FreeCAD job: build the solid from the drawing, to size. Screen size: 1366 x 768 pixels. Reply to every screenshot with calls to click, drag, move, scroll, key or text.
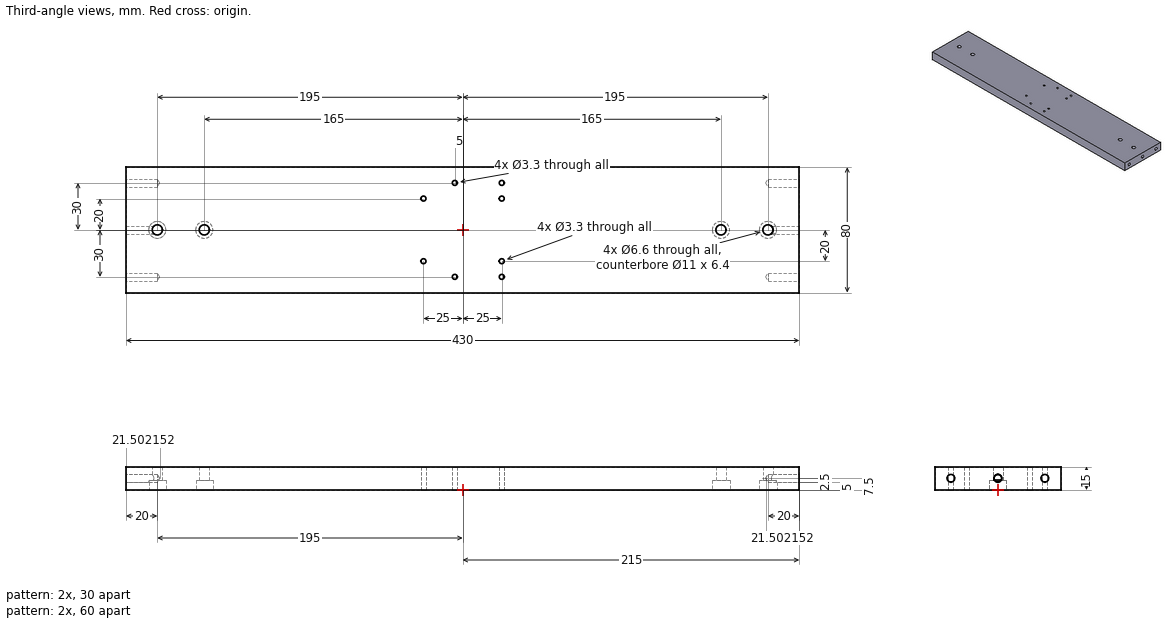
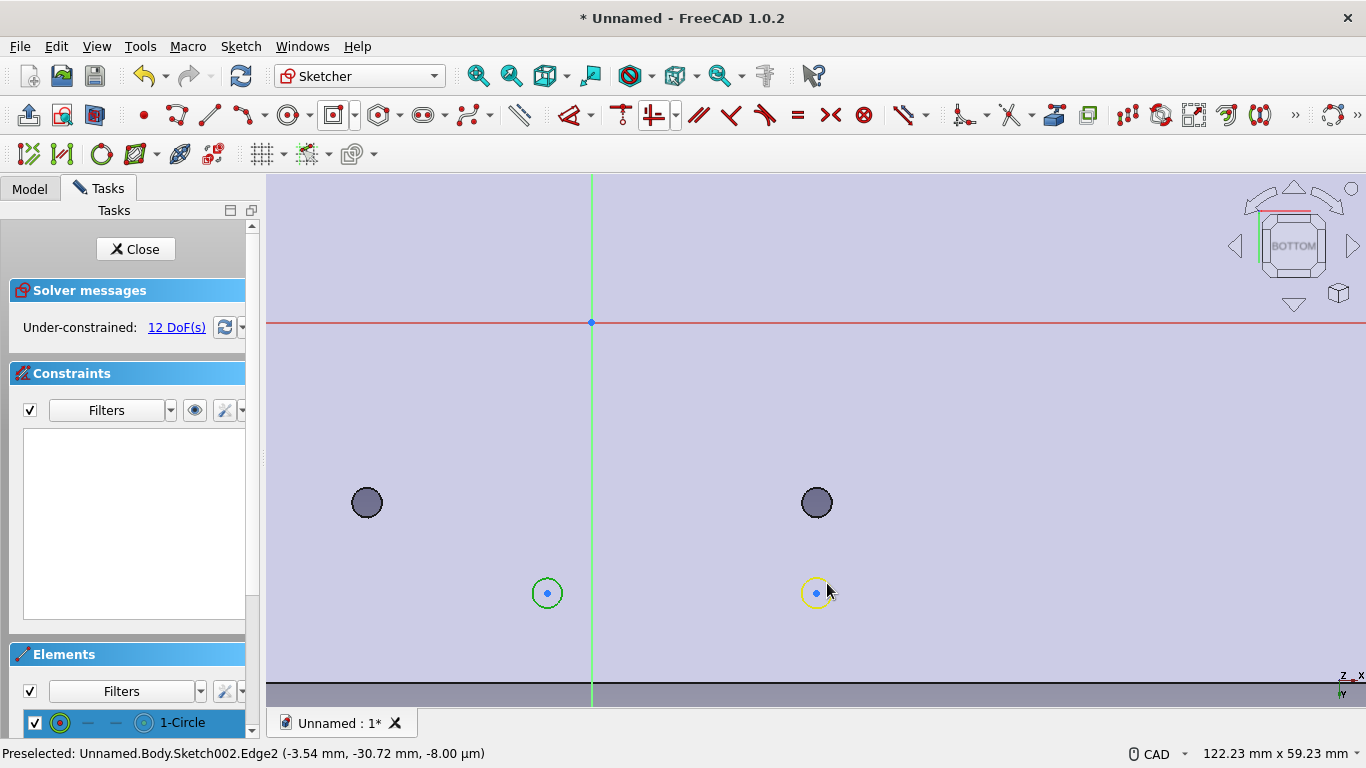
click(827, 582)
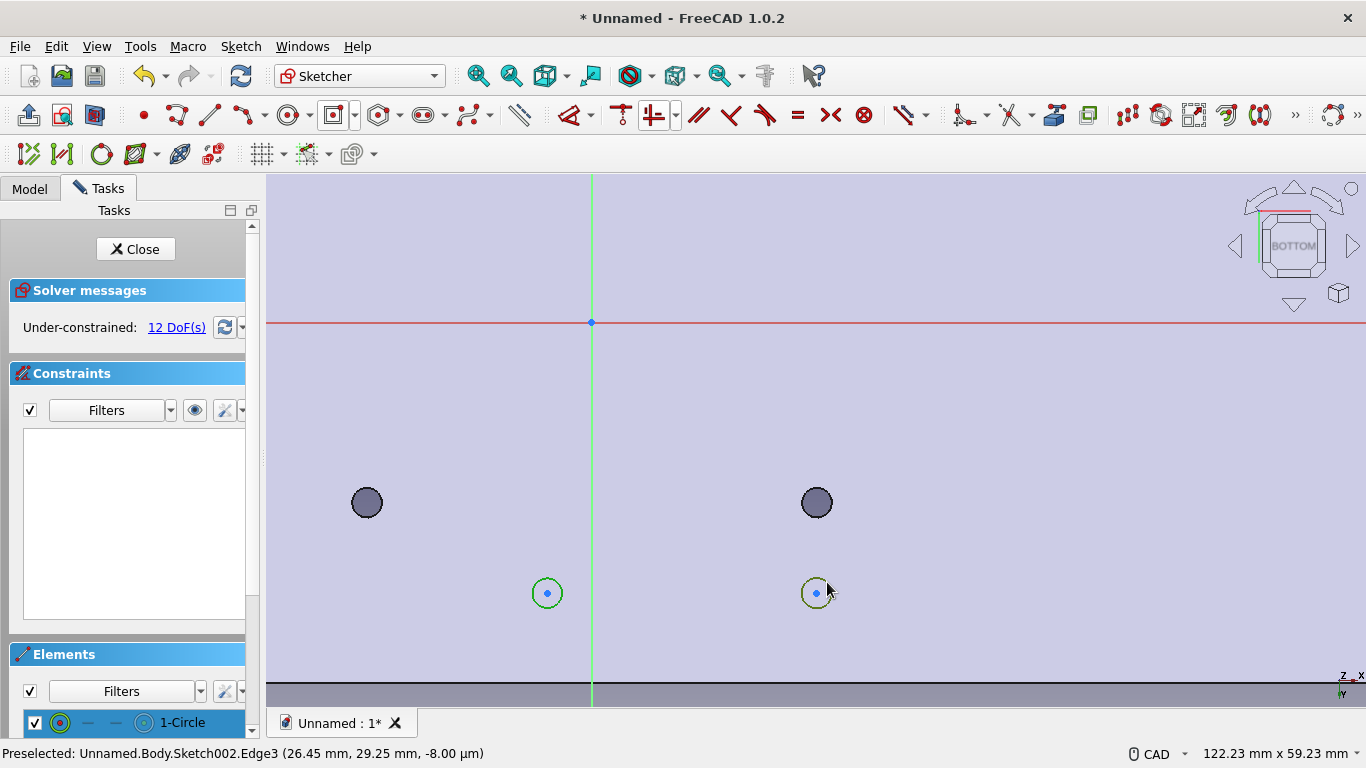
scroll(827, 584, down, 3)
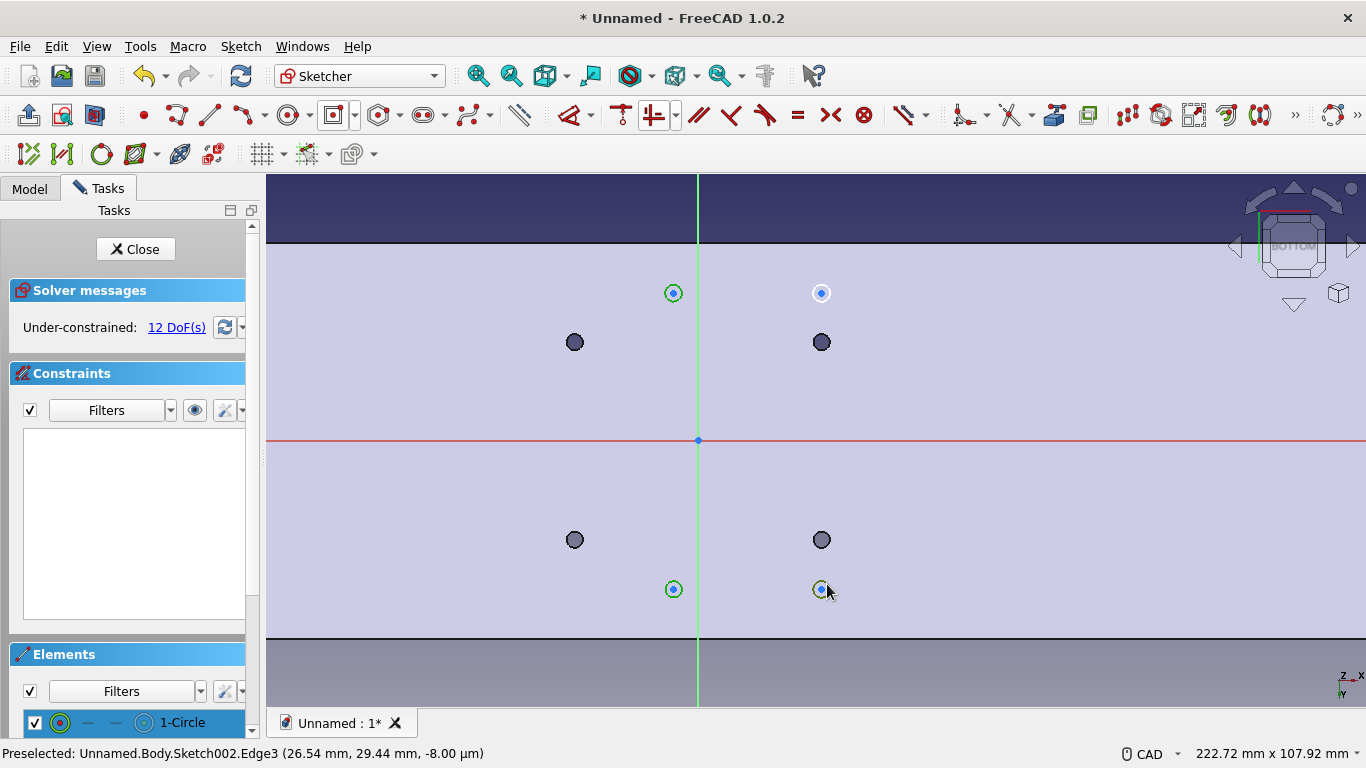
scroll(828, 287, up, 3)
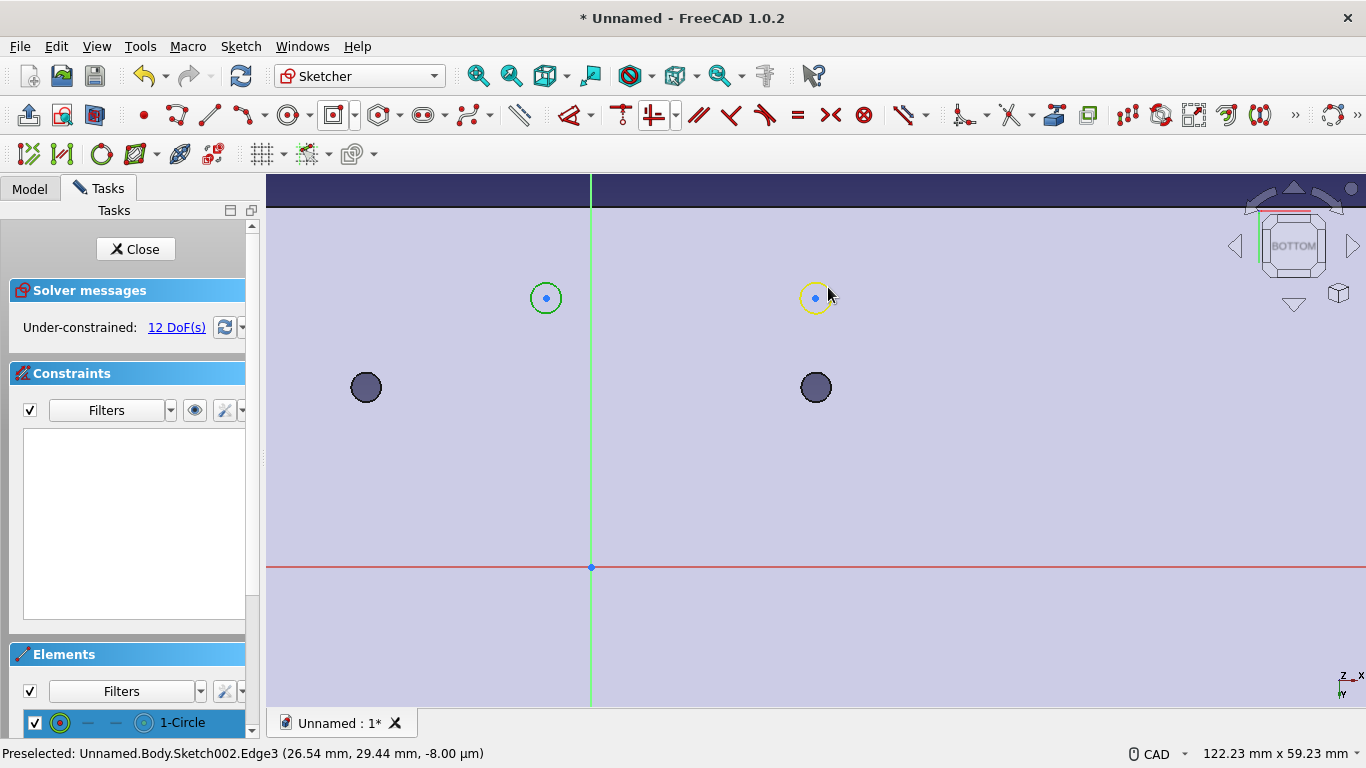
click(827, 287)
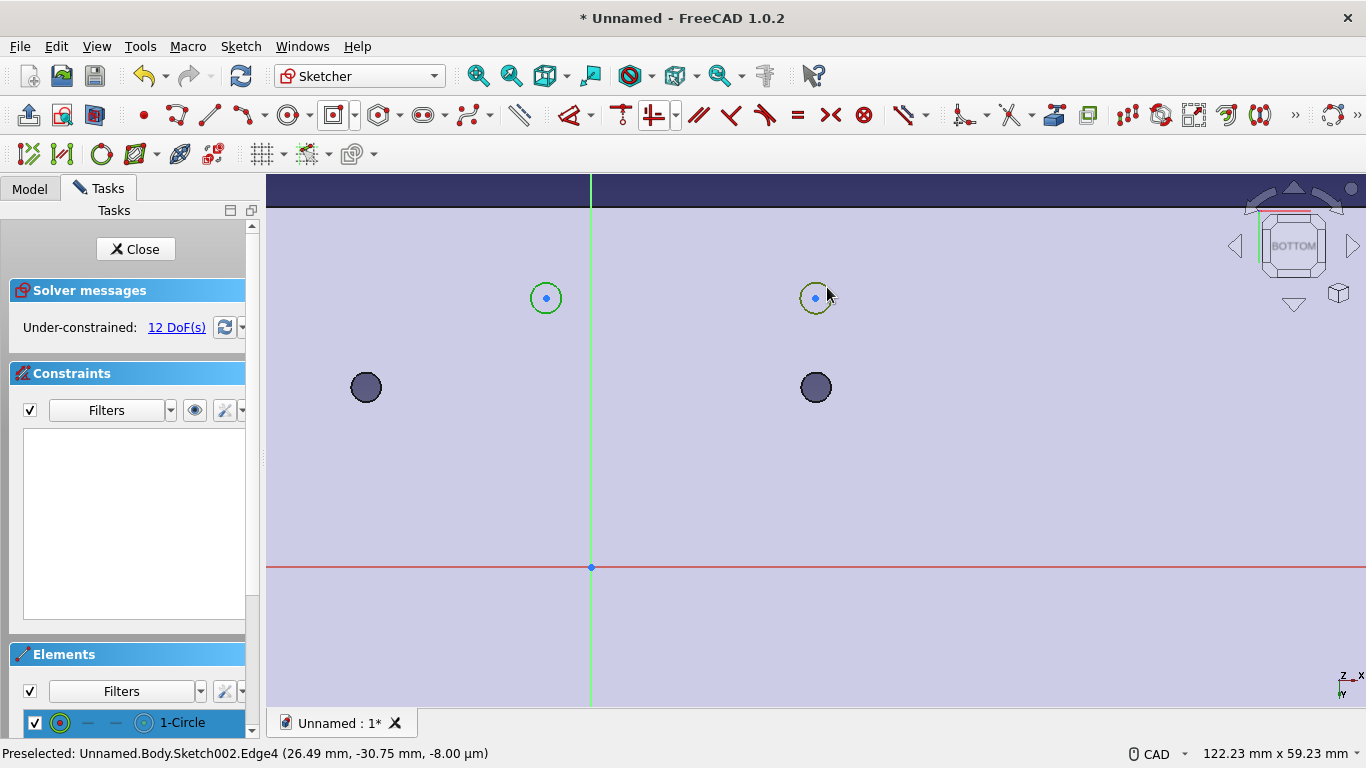
click(798, 116)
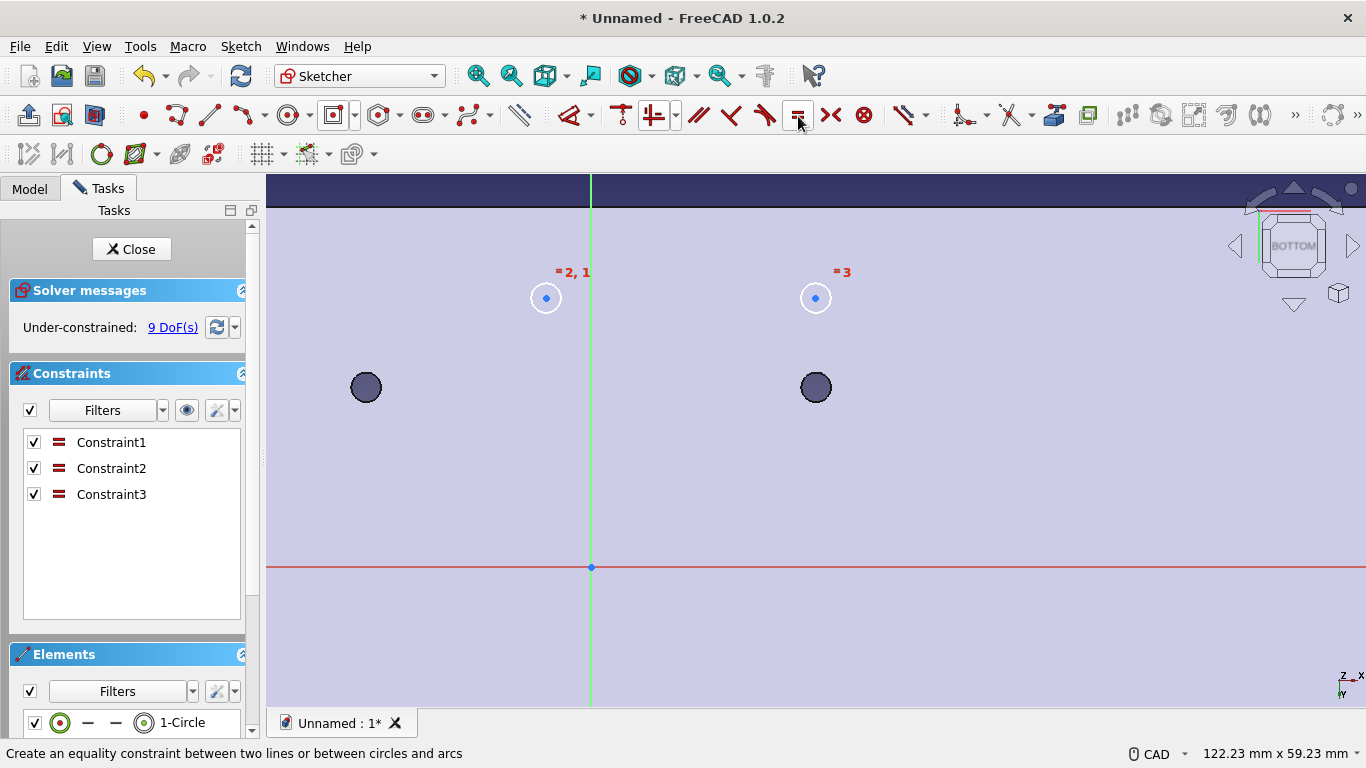
scroll(828, 286, down, 3)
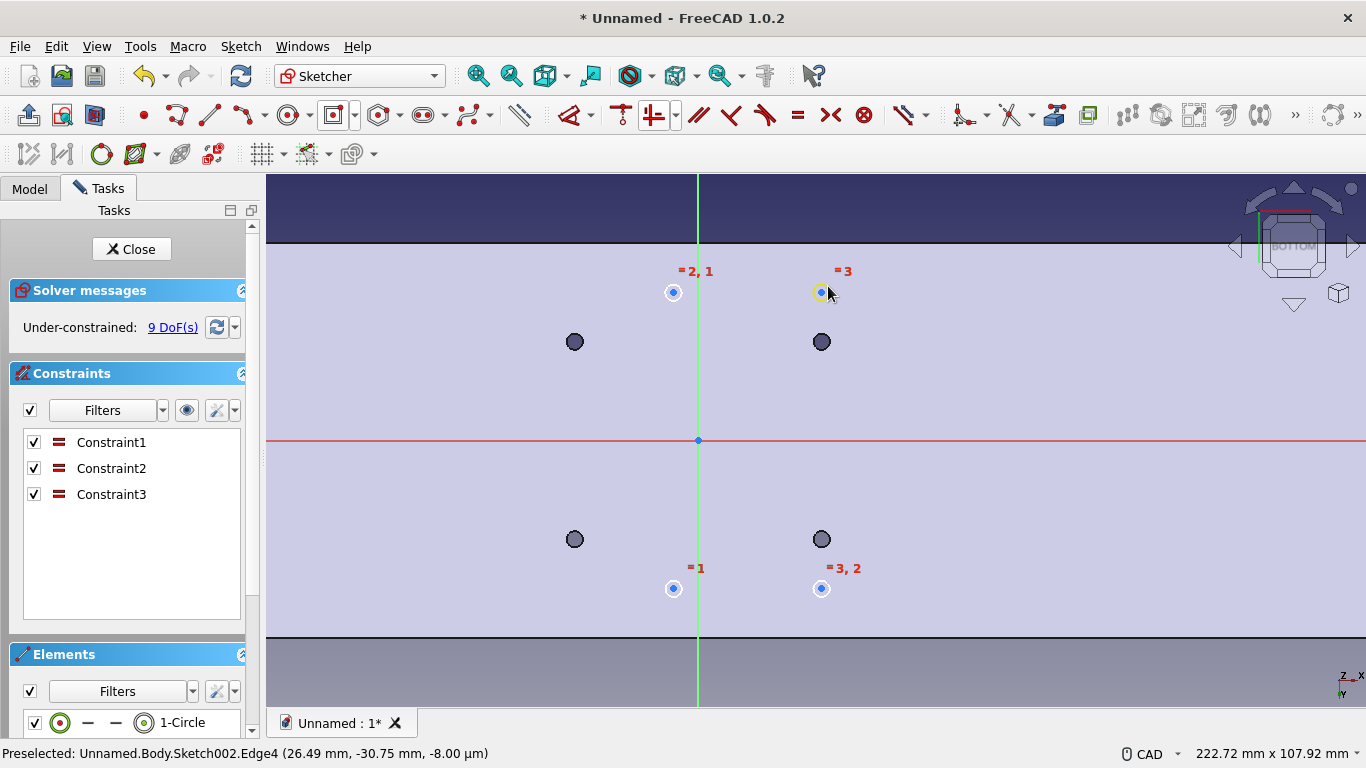
click(674, 589)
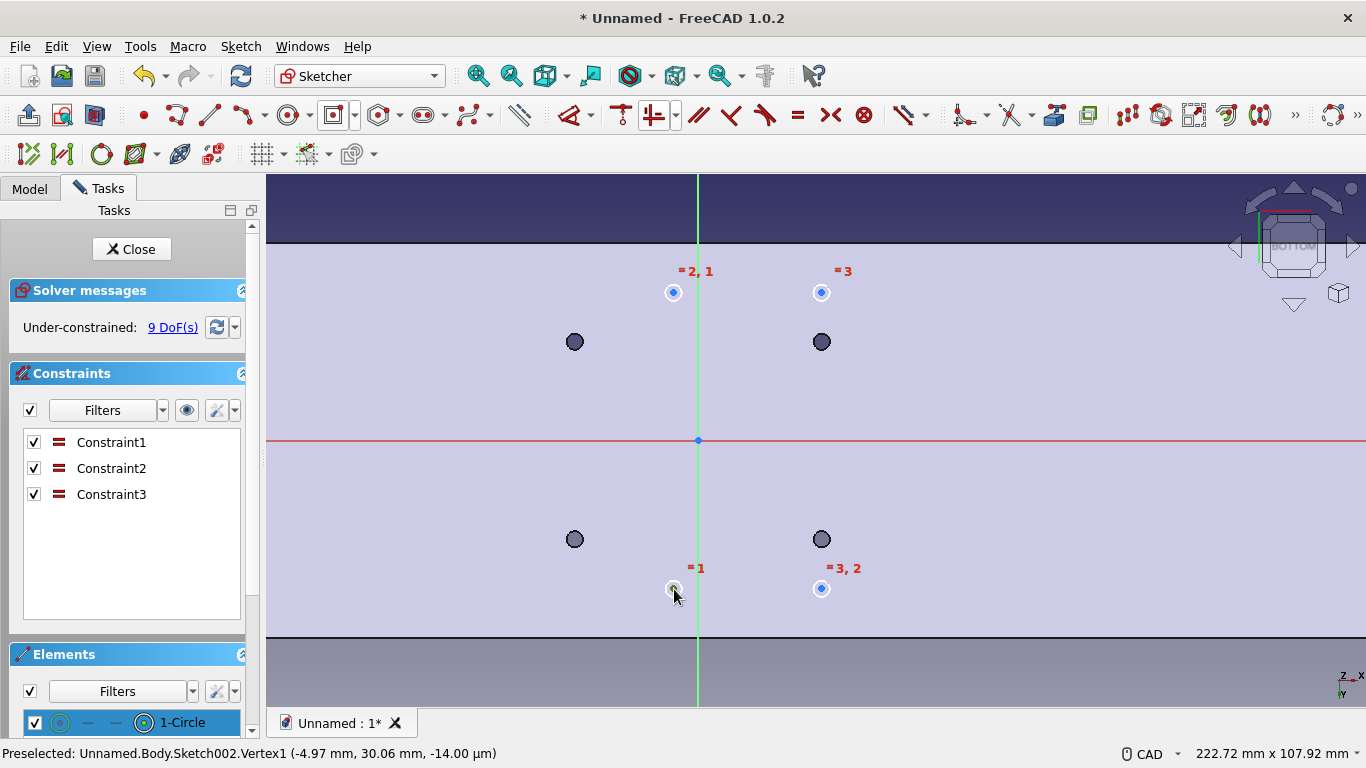
click(674, 293)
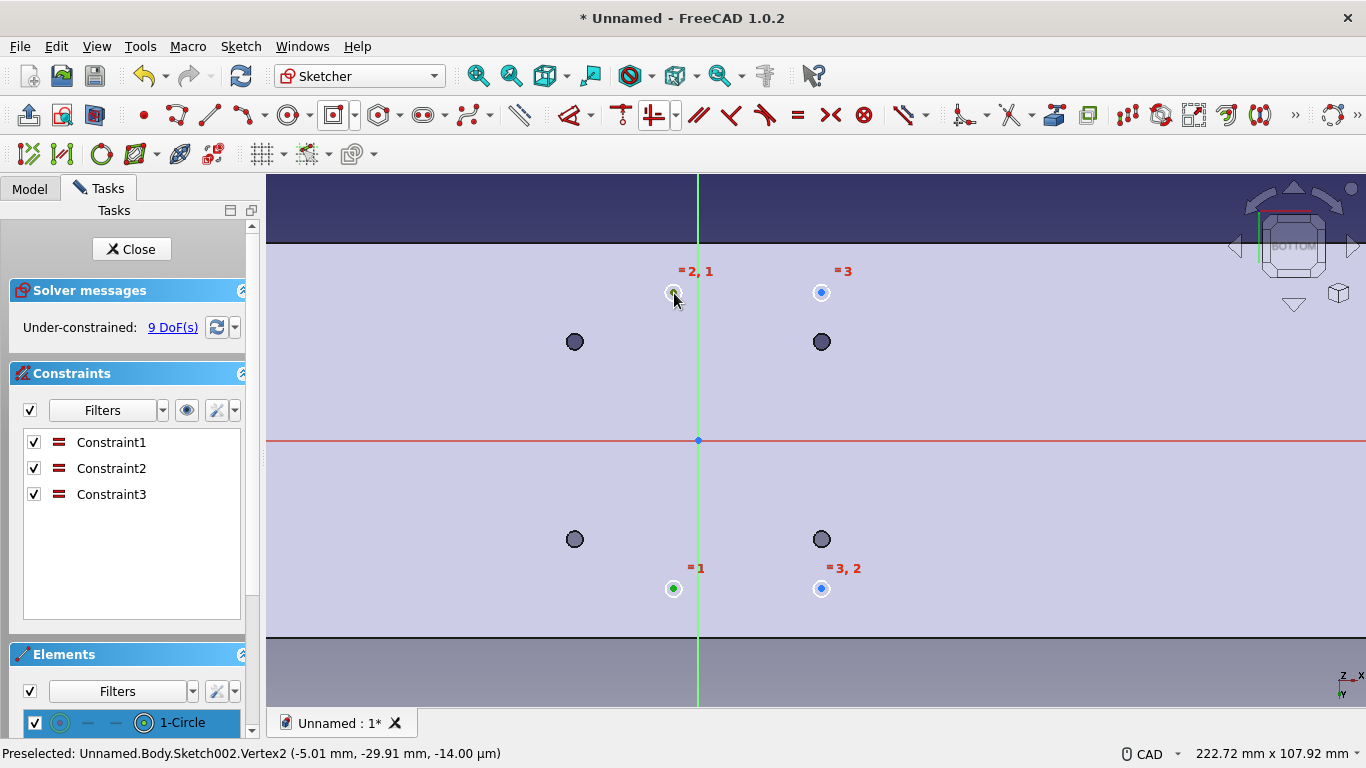
click(676, 116)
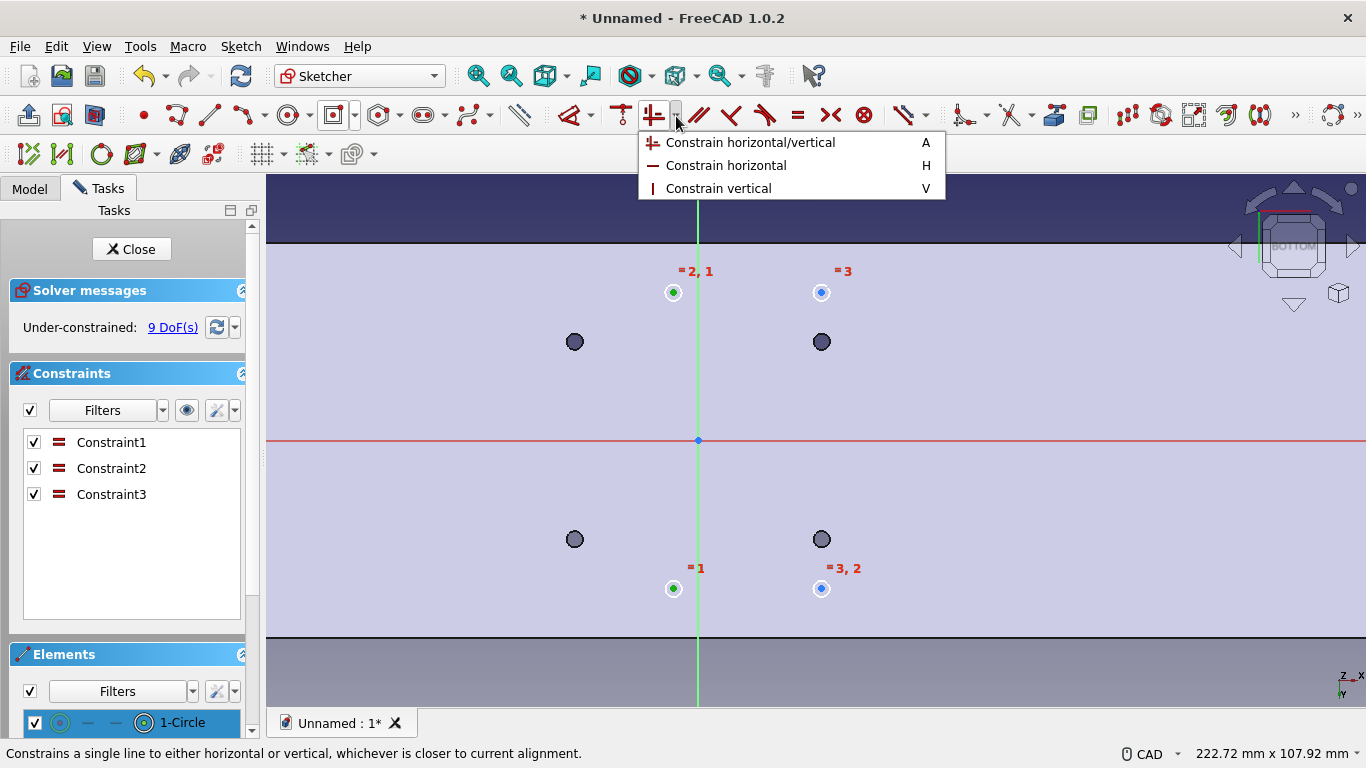
click(792, 188)